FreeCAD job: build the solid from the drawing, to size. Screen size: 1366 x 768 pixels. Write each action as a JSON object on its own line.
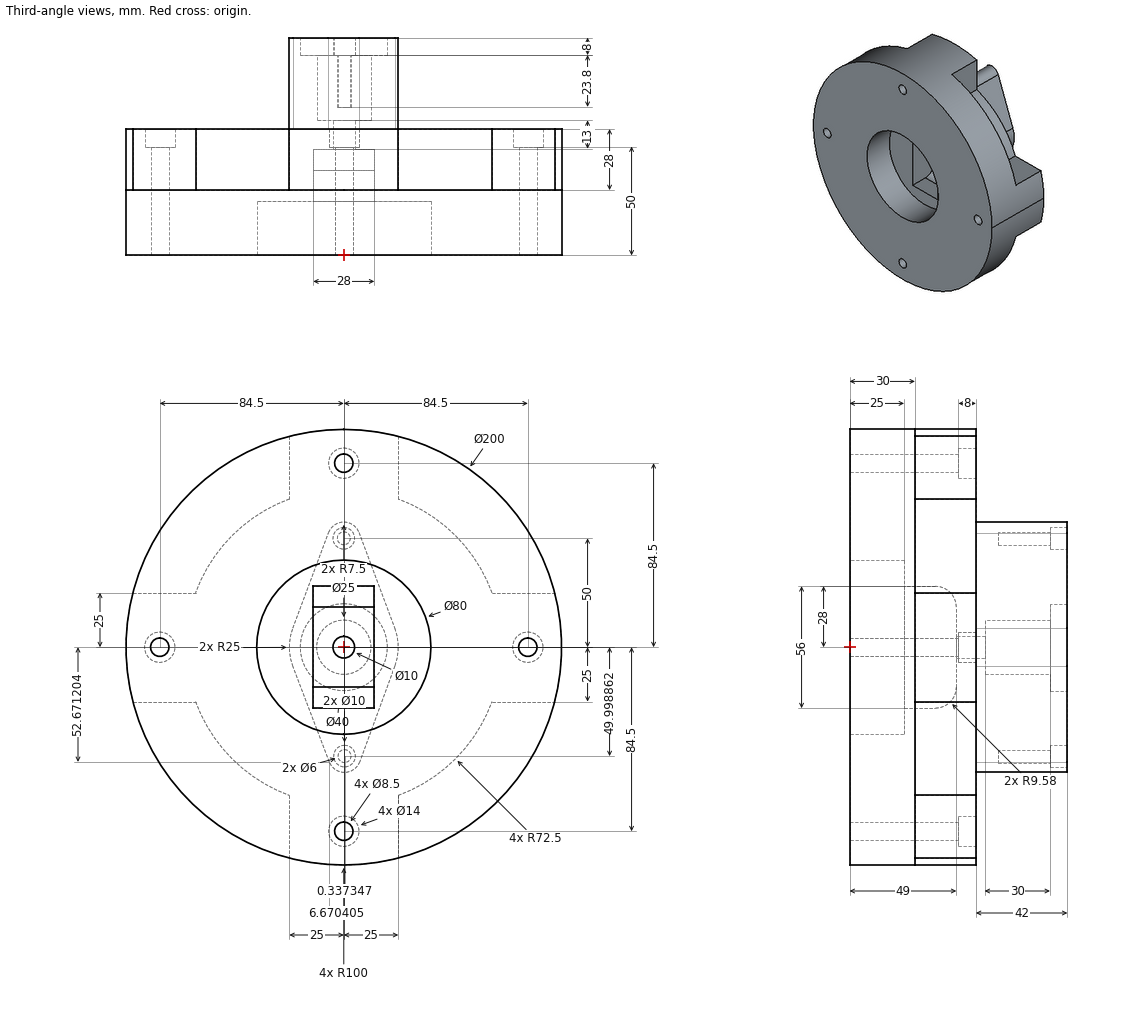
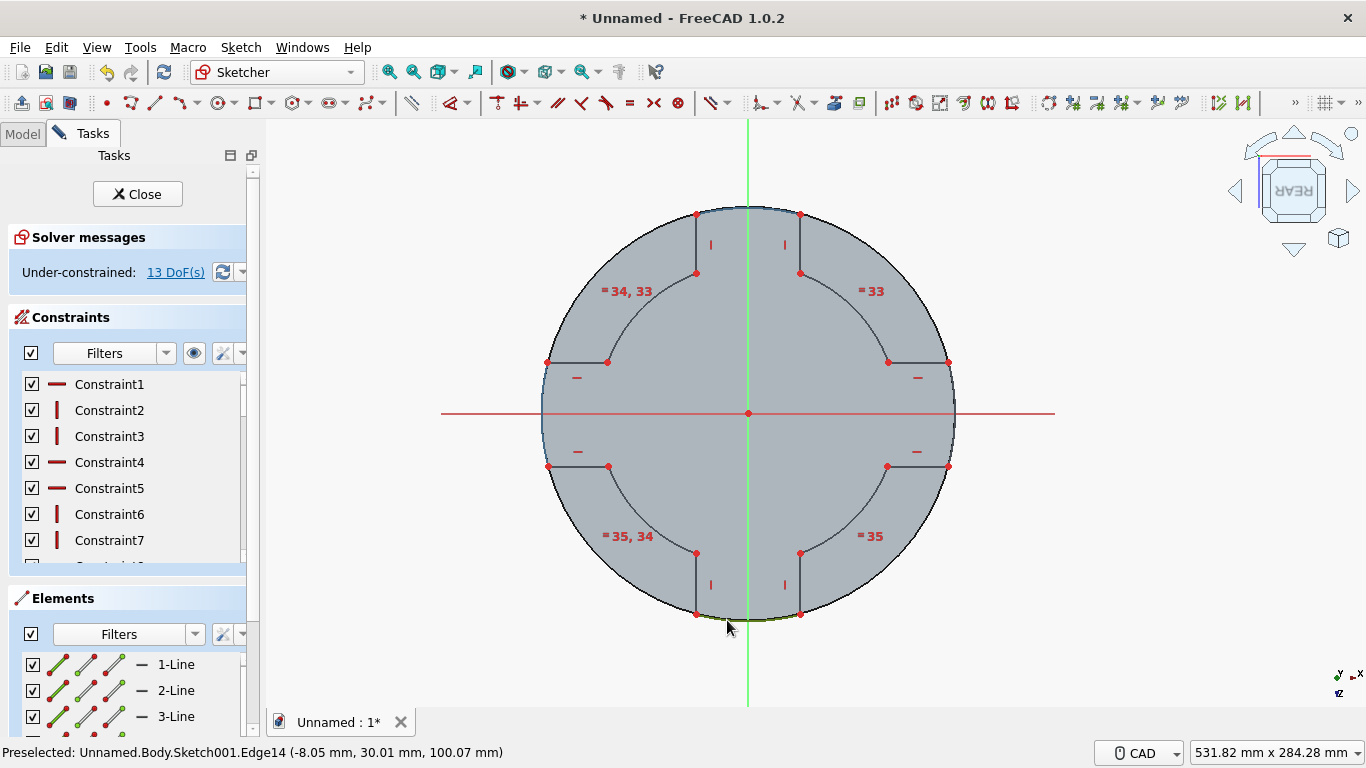
{"action": "left_click", "coordinate": [954, 436]}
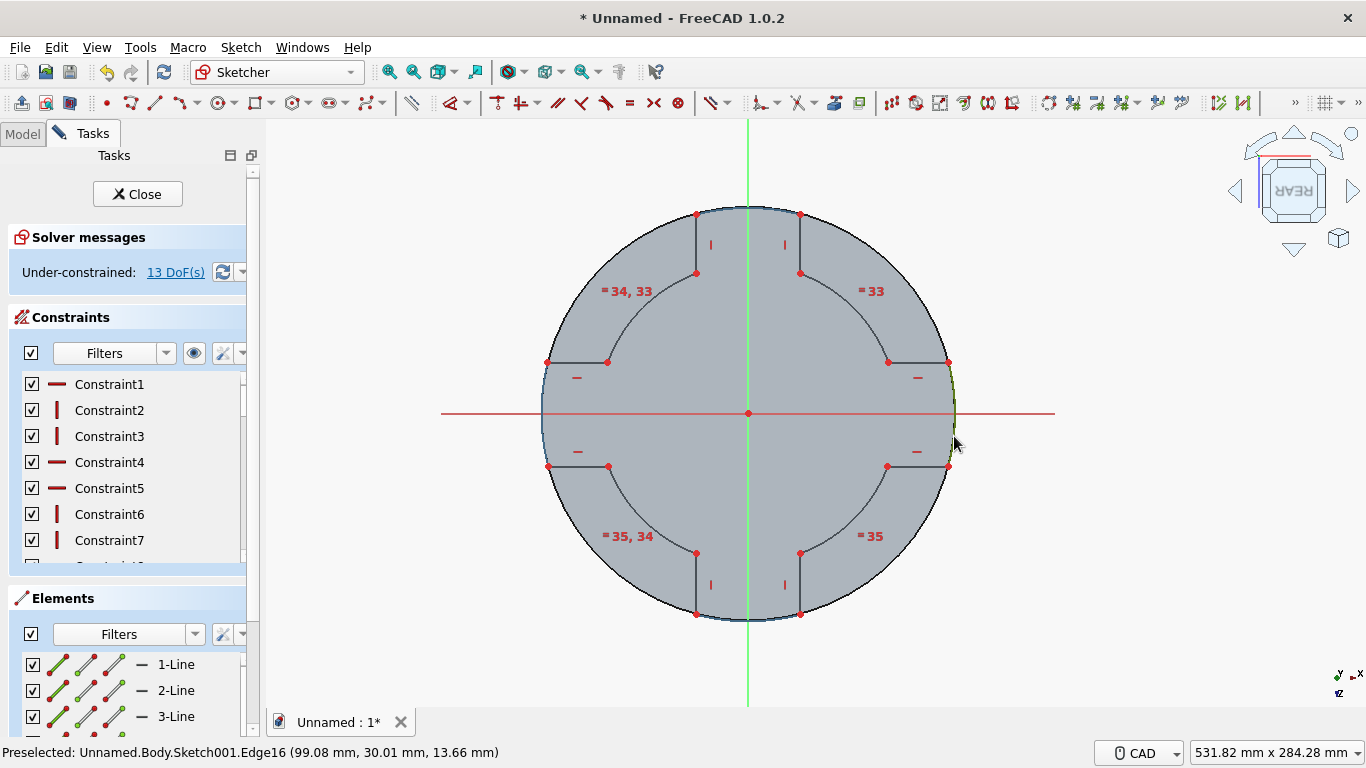
{"action": "key", "text": "e"}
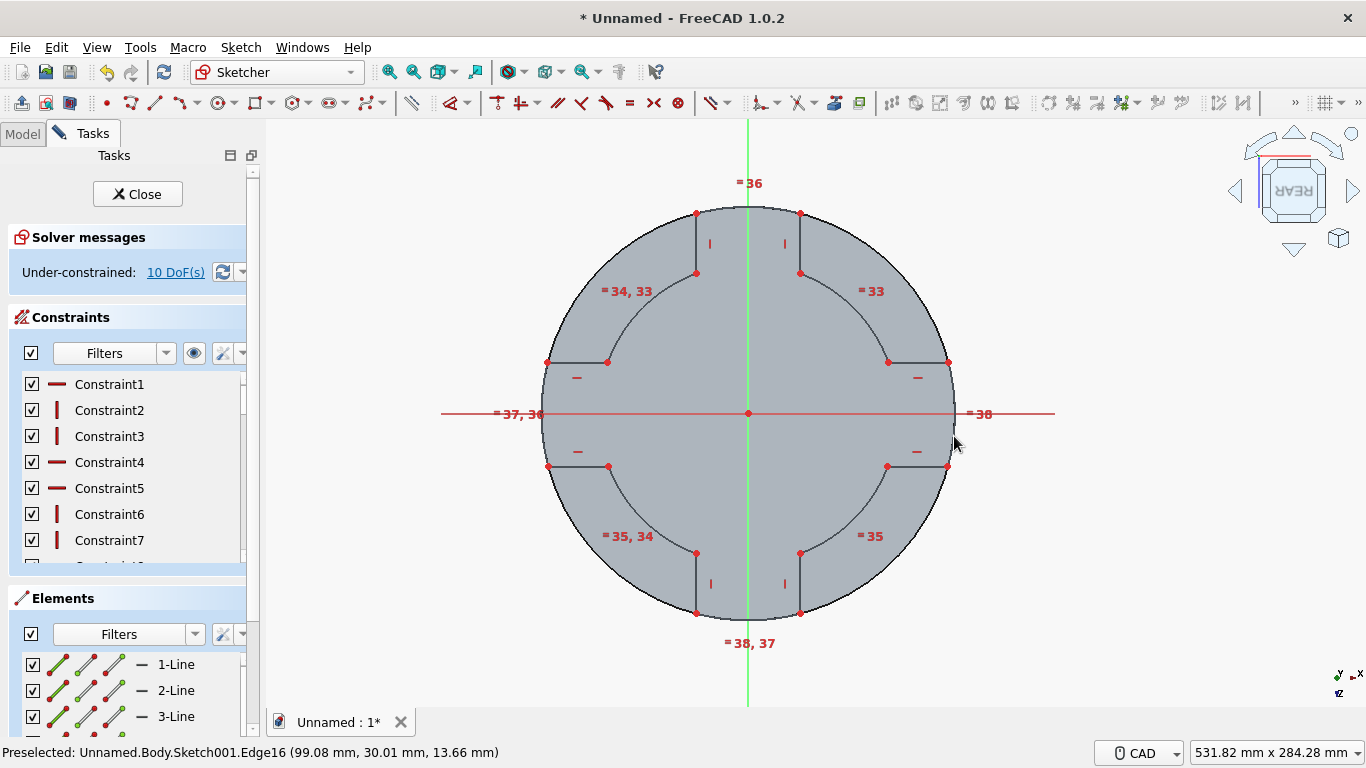
{"action": "left_click", "coordinate": [450, 104]}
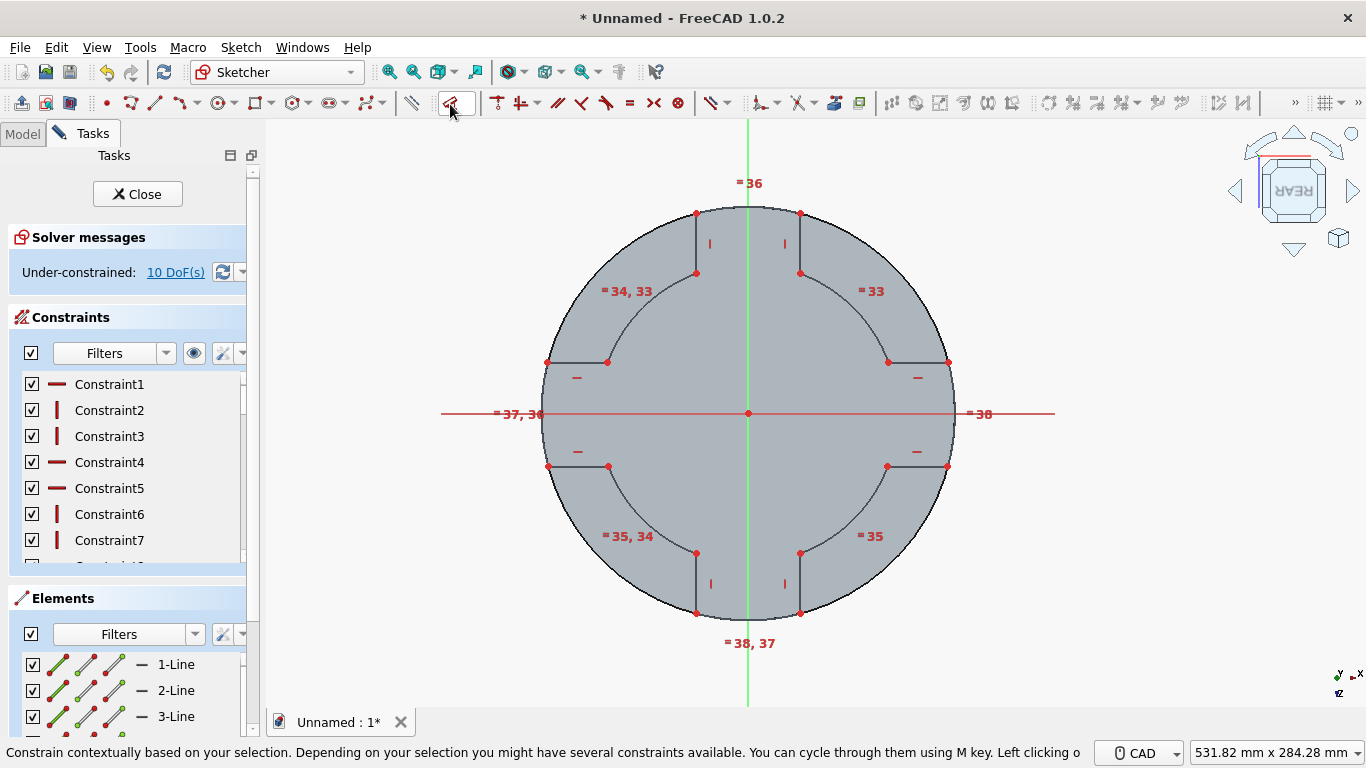
{"action": "left_click", "coordinate": [871, 328]}
{"action": "left_click", "coordinate": [897, 310]}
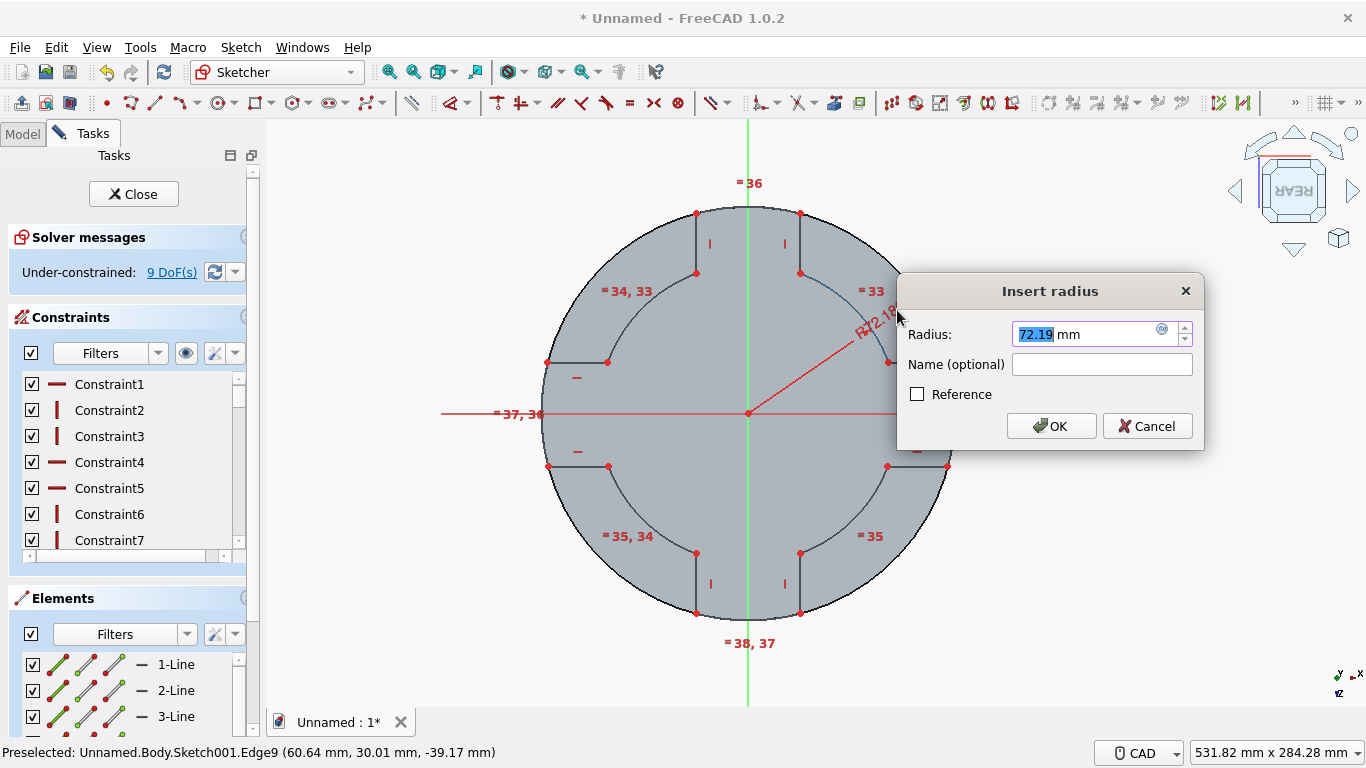
{"action": "type", "text": "72.5"}
{"action": "key", "text": "Return"}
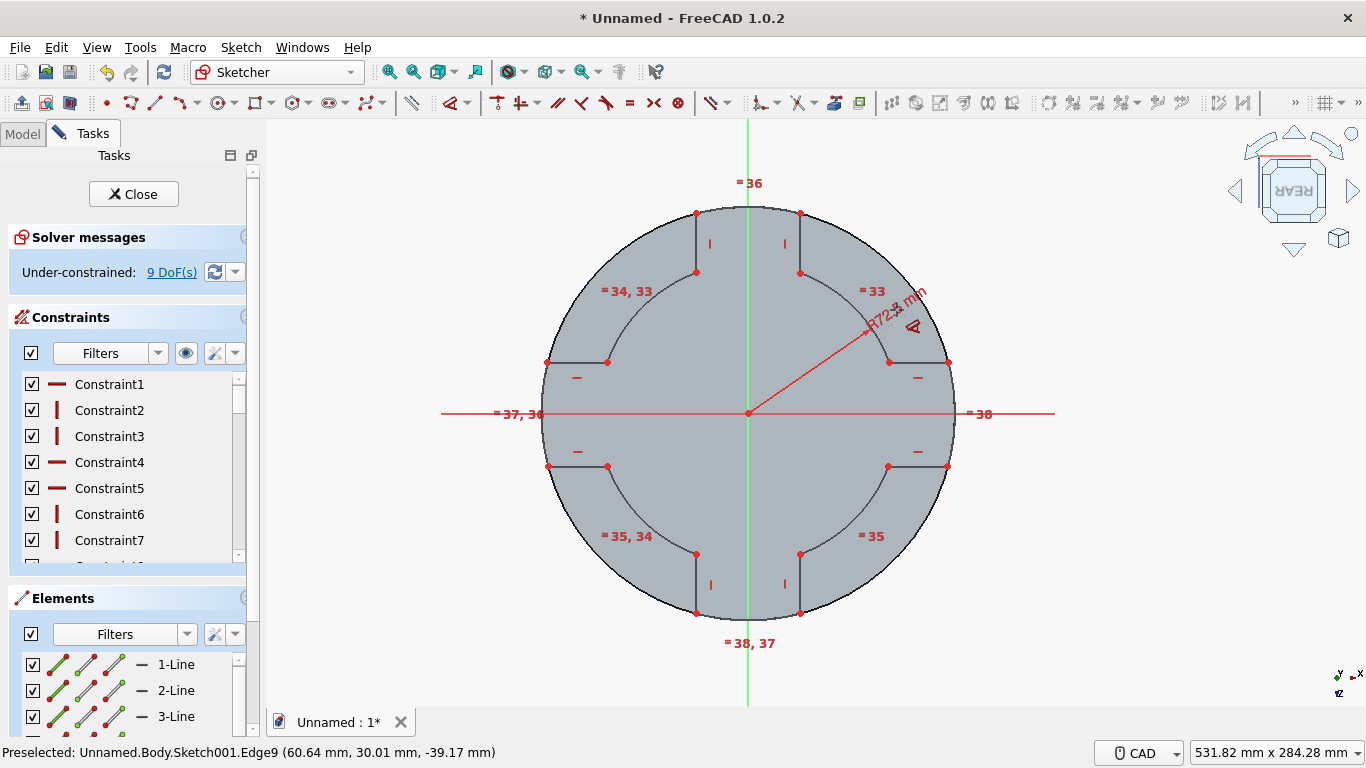
{"action": "left_click", "coordinate": [769, 208]}
{"action": "left_click", "coordinate": [772, 176]}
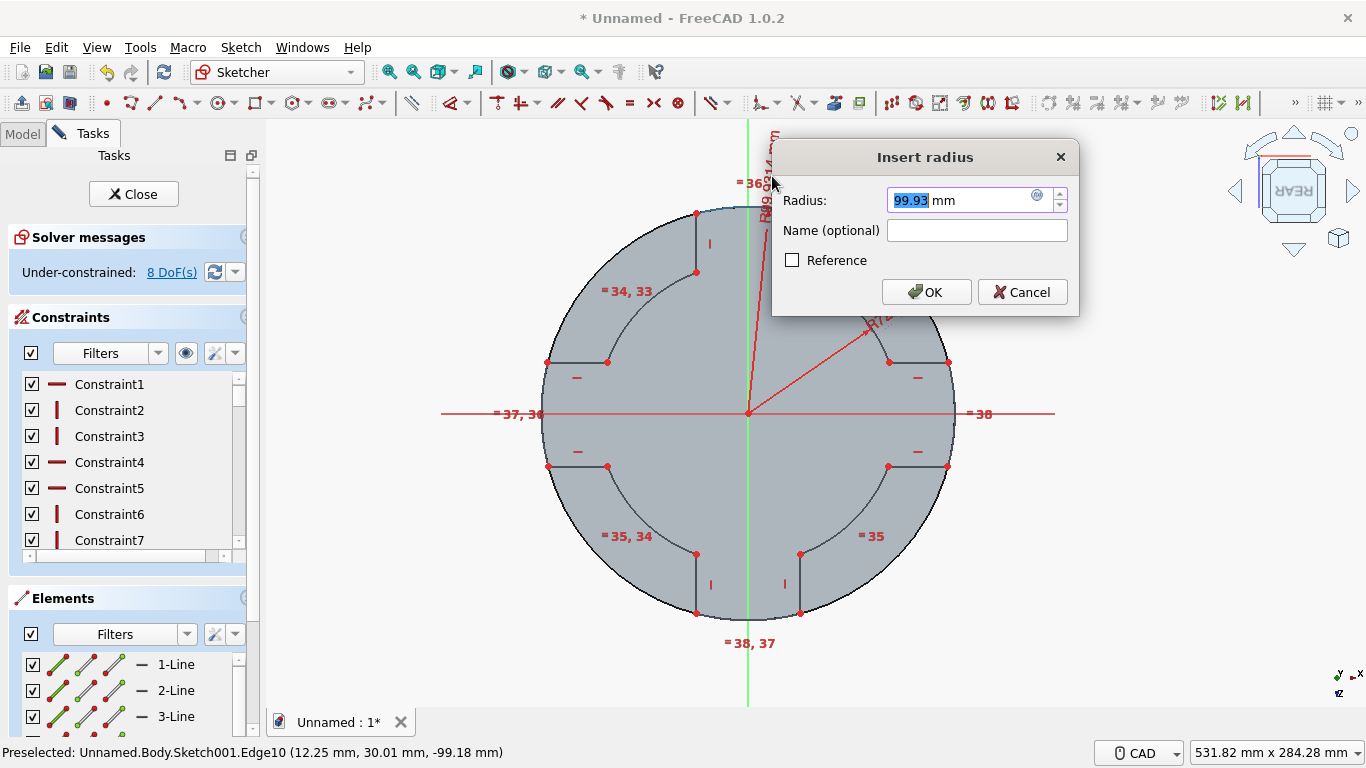
{"action": "type", "text": "100"}
{"action": "key", "text": "Return"}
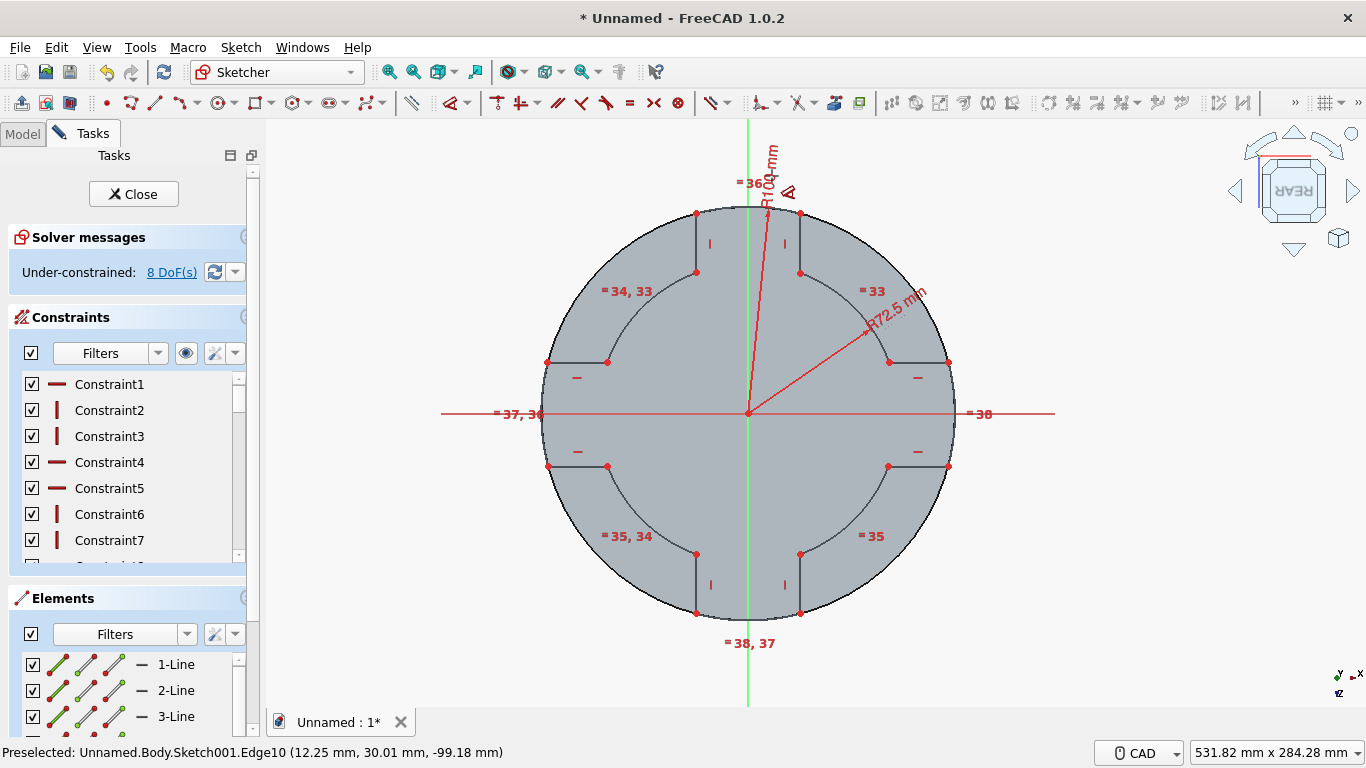
{"action": "left_click", "coordinate": [949, 363]}
{"action": "left_click", "coordinate": [983, 388]}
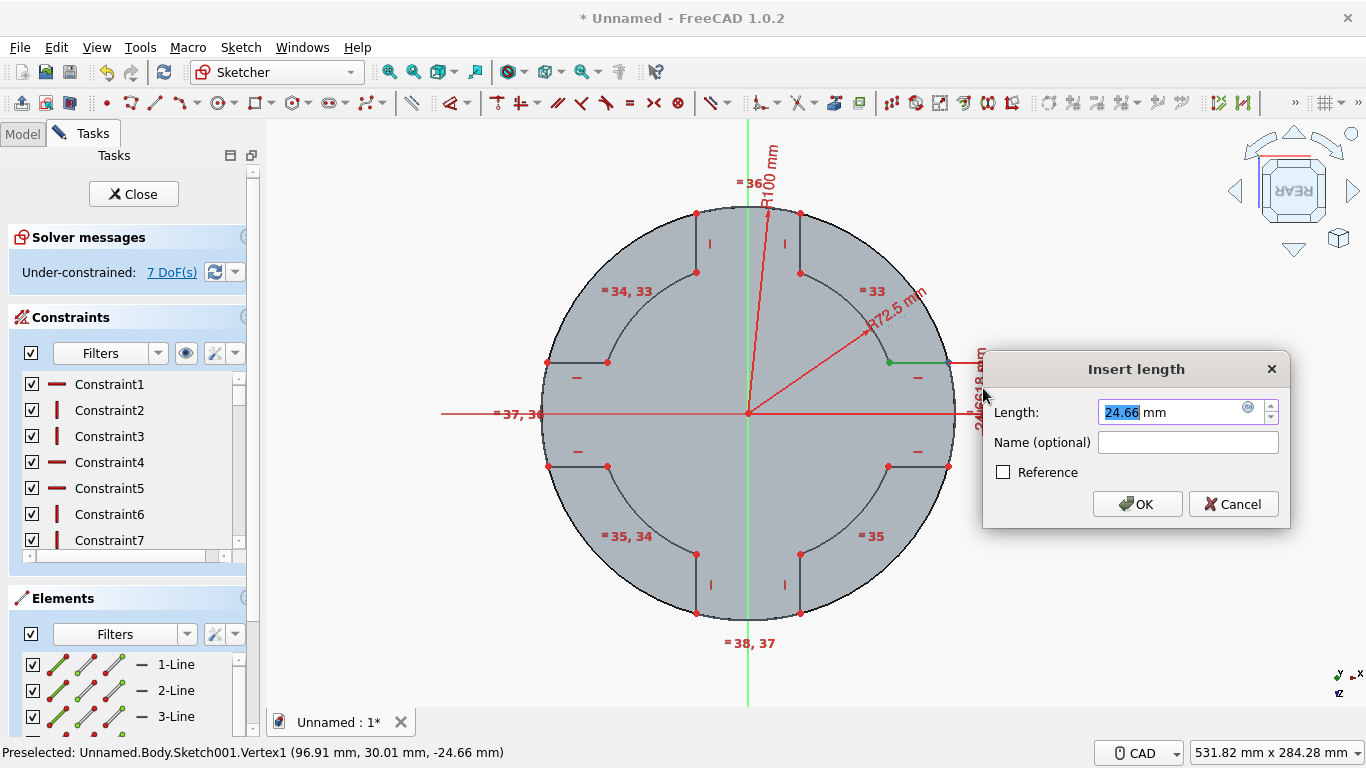
{"action": "type", "text": "25"}
{"action": "key", "text": "Return"}